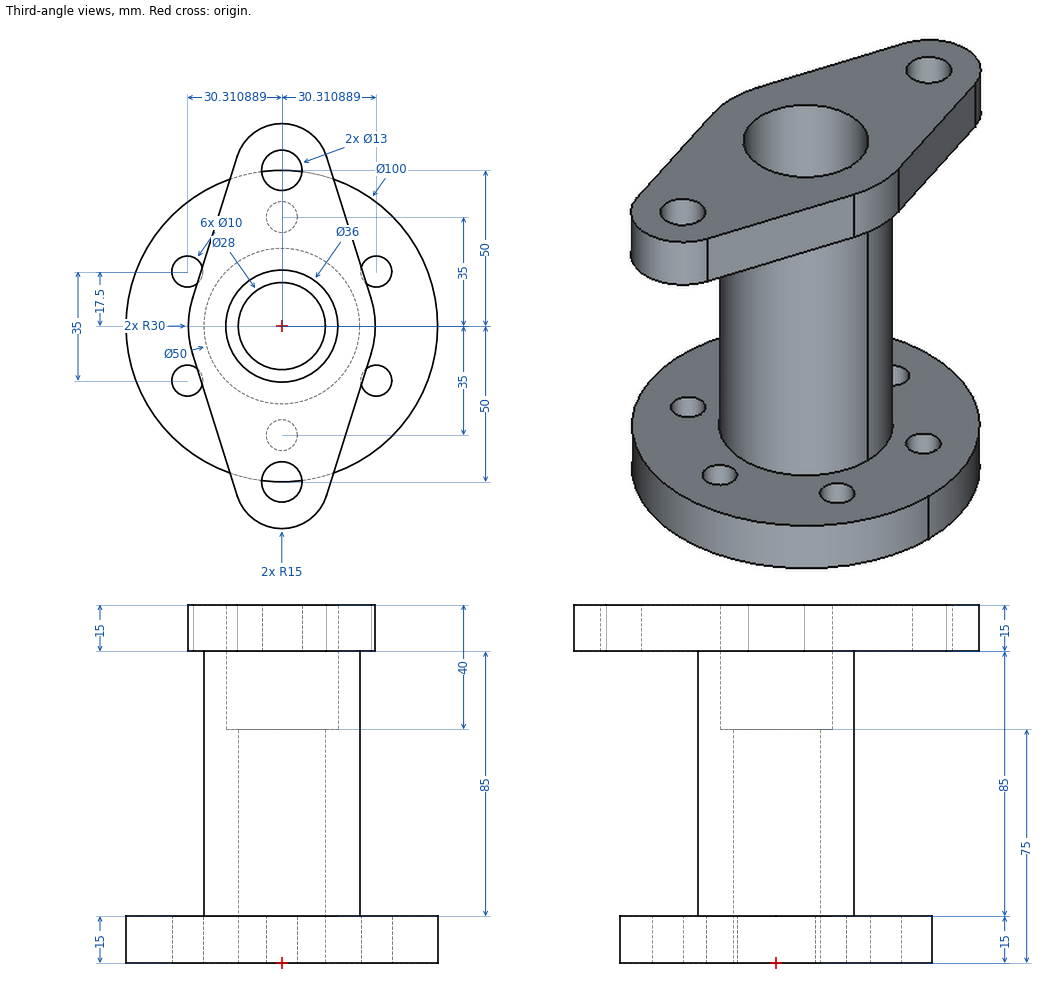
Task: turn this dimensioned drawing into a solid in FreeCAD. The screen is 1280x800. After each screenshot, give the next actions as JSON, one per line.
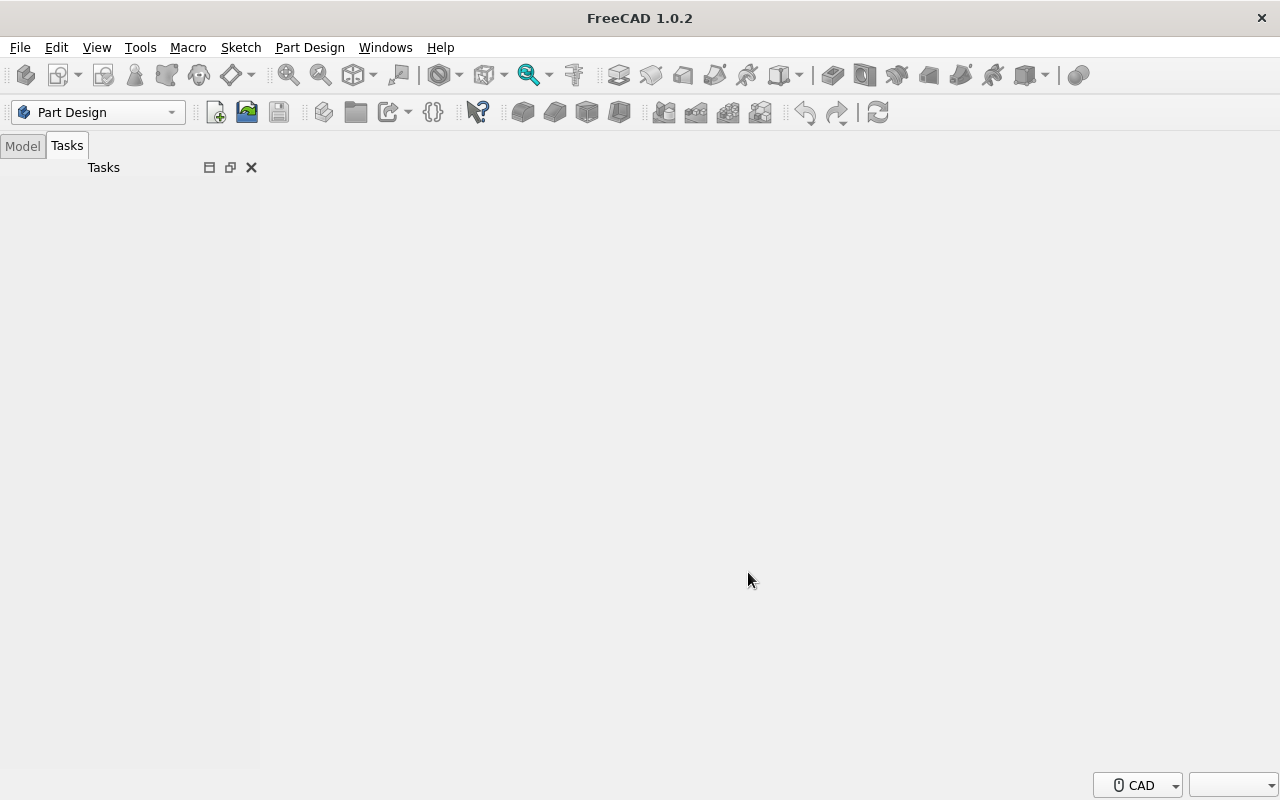
{"action": "key", "text": "ctrl+n"}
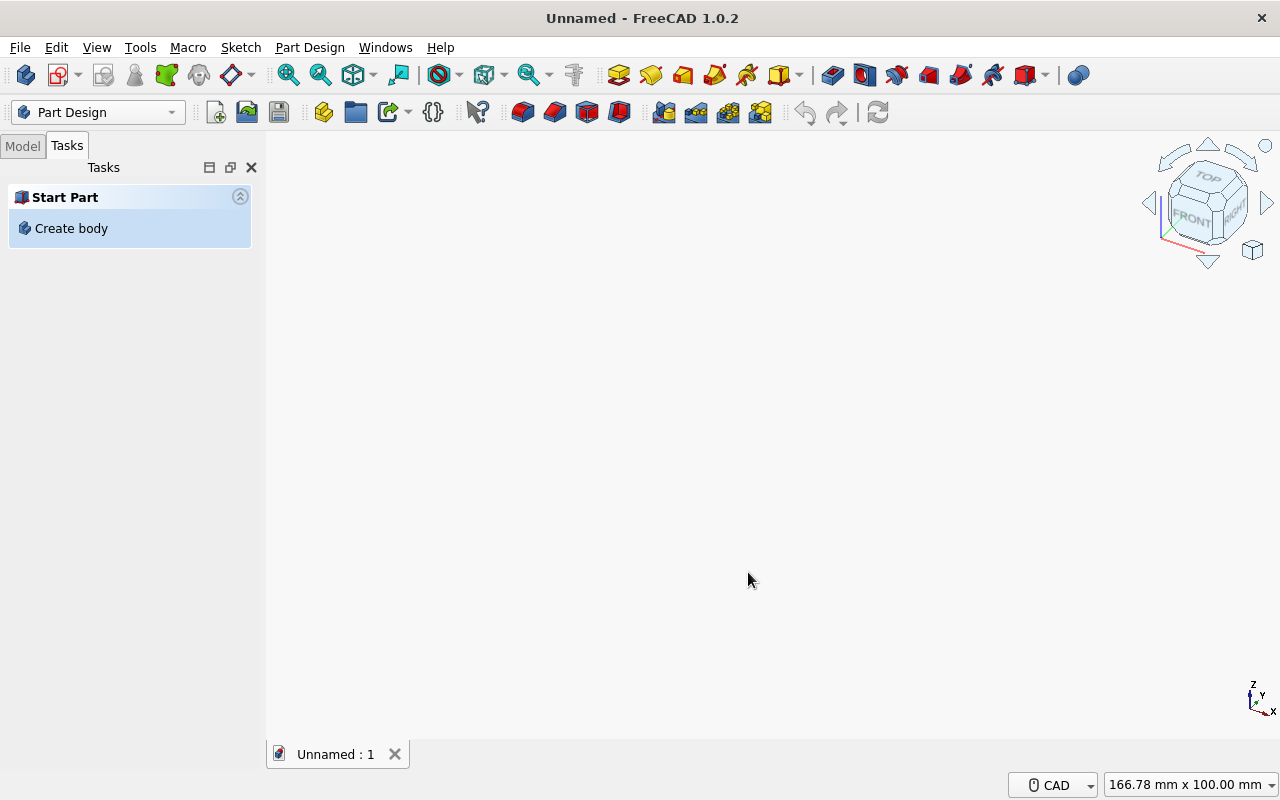
{"action": "left_click", "coordinate": [58, 76]}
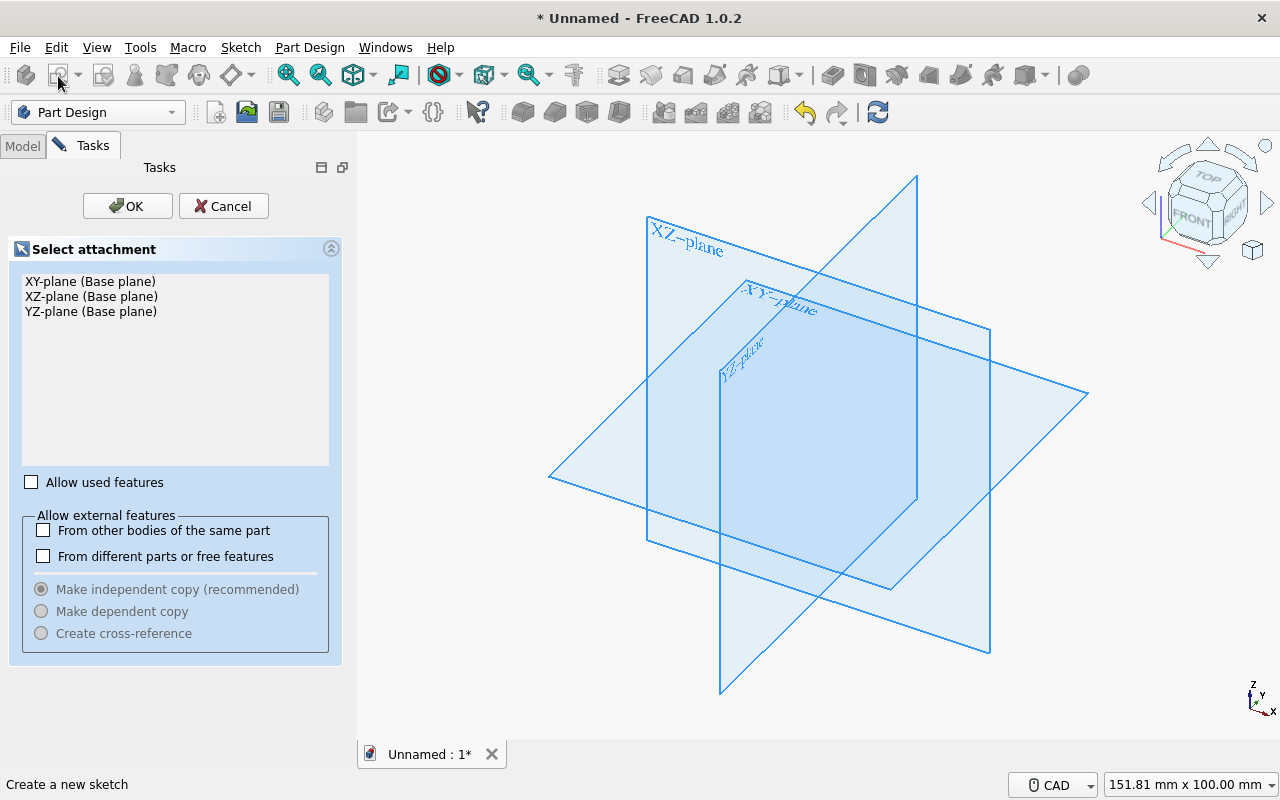
{"action": "left_click", "coordinate": [82, 282]}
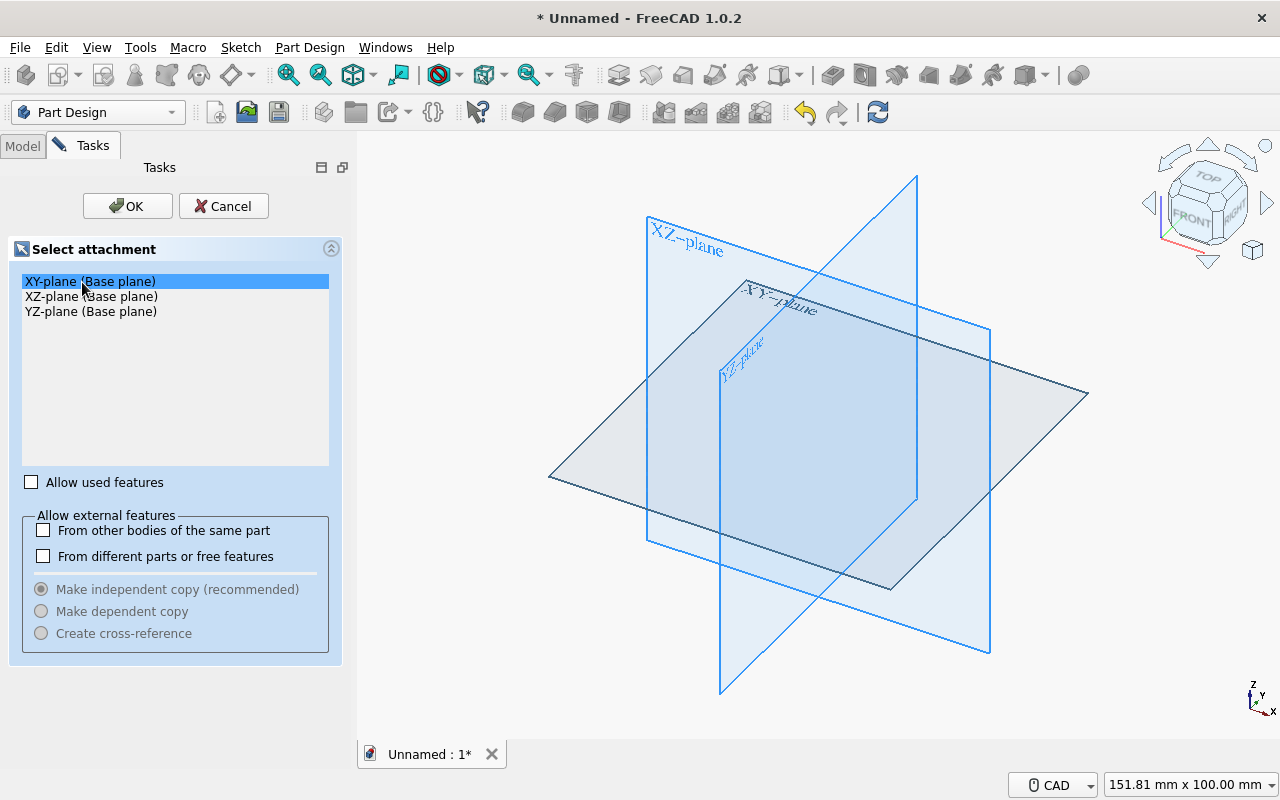
{"action": "left_click", "coordinate": [128, 206]}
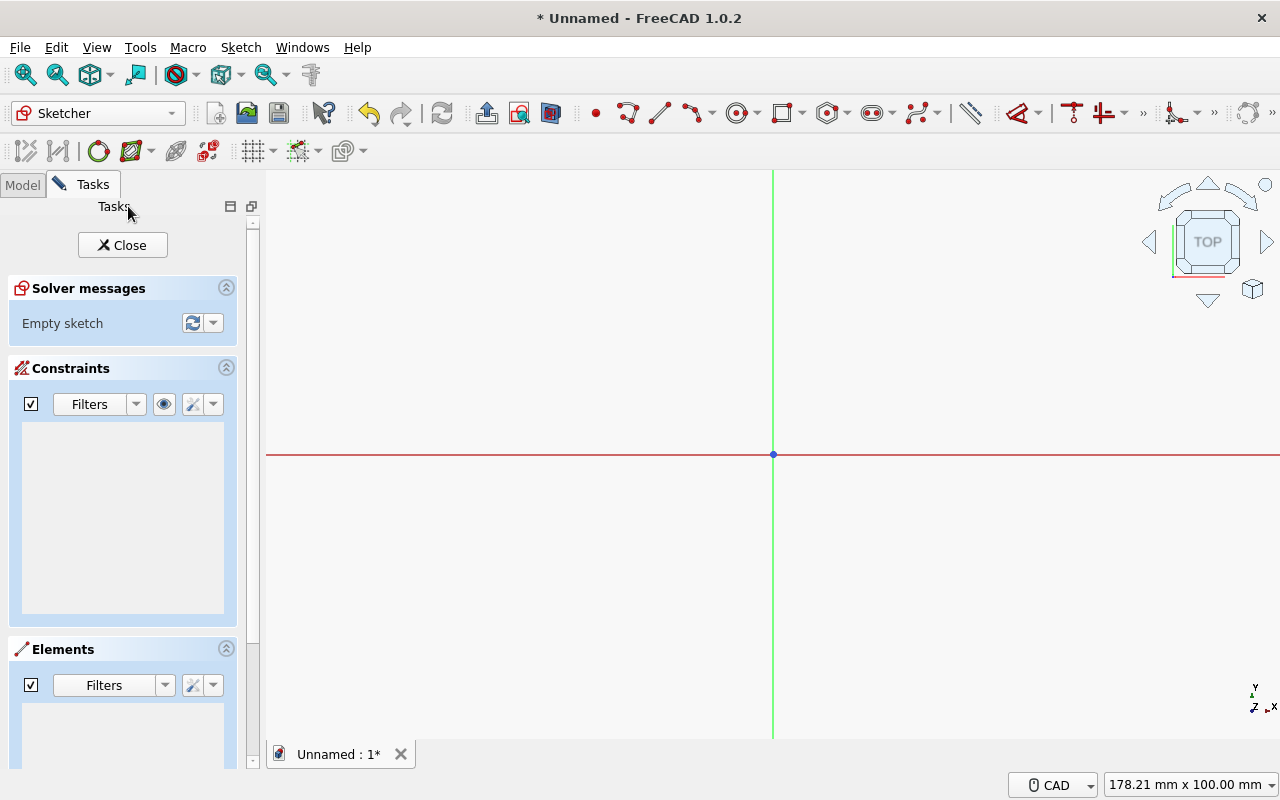
{"action": "scroll", "coordinate": [565, 455], "scroll_direction": "down", "scroll_amount": 2}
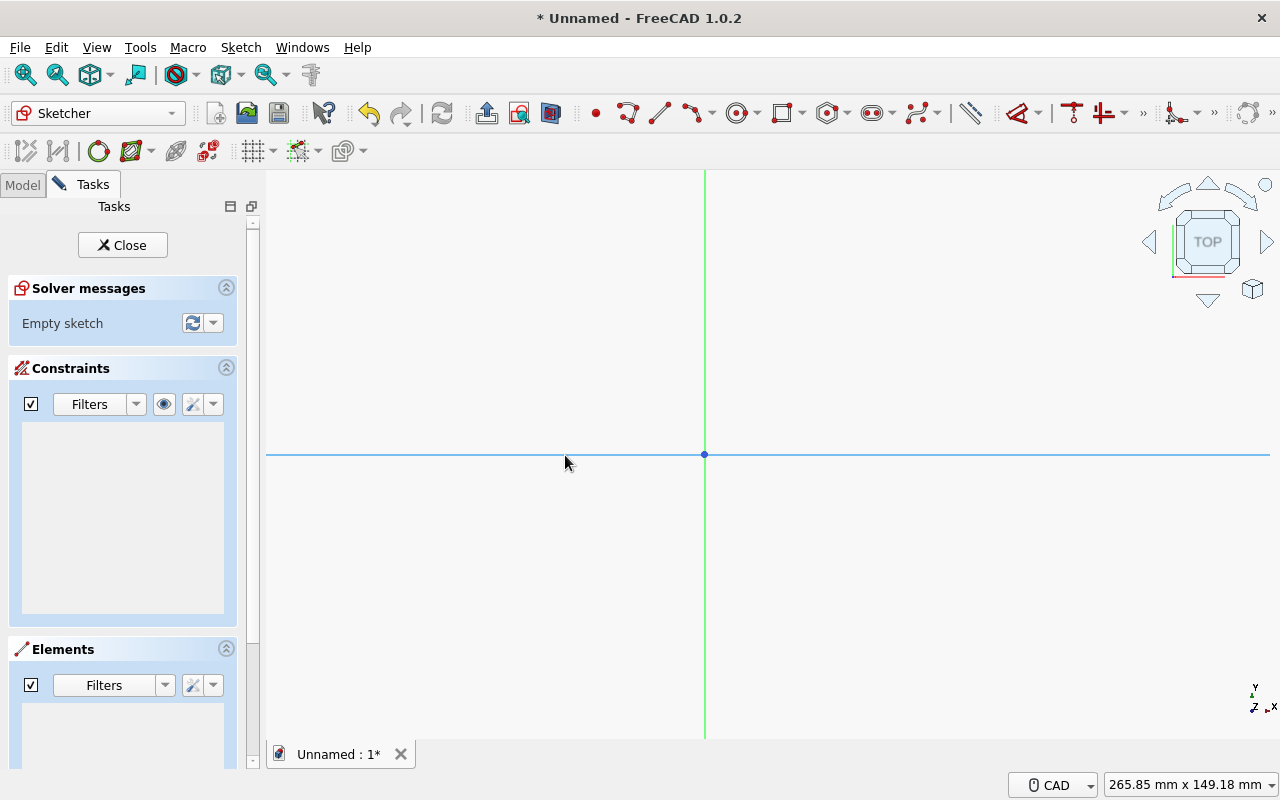
{"action": "left_click", "coordinate": [738, 114]}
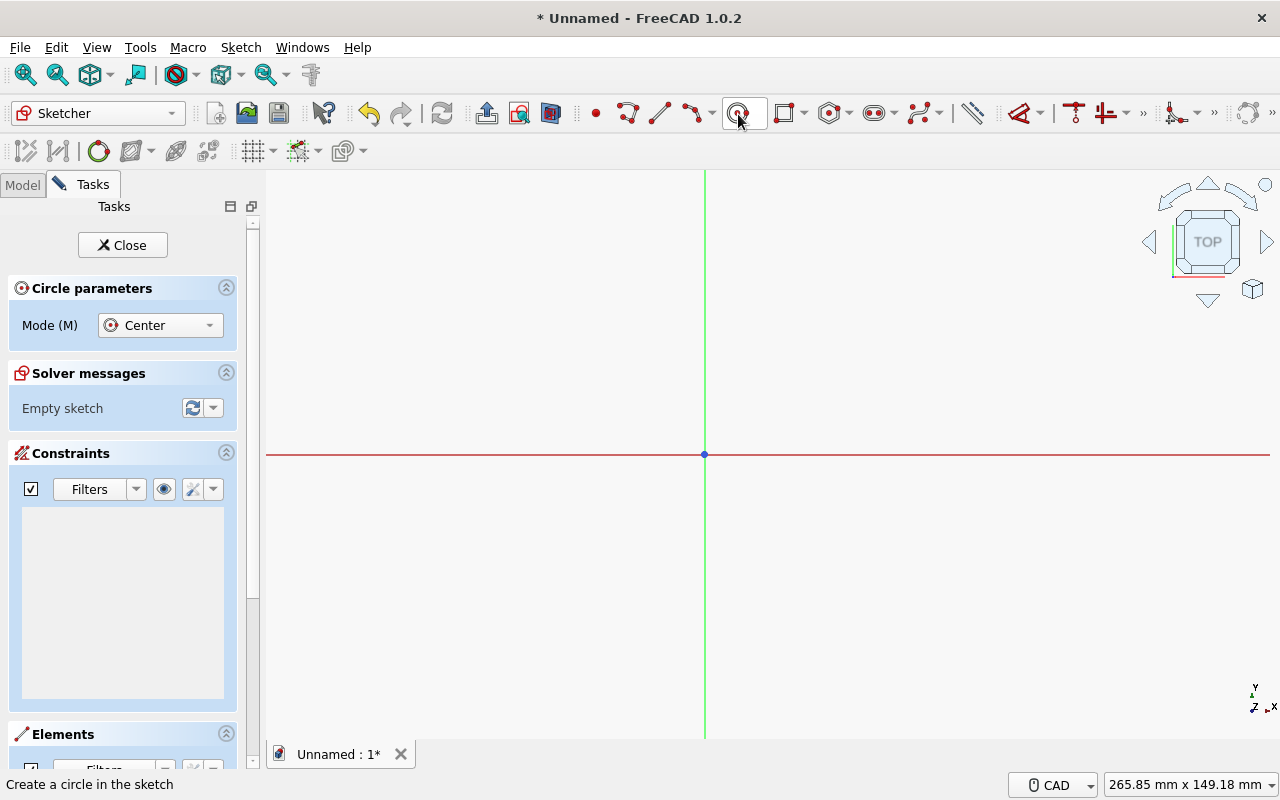
{"action": "left_click", "coordinate": [705, 455]}
{"action": "mouse_move", "coordinate": [839, 320]}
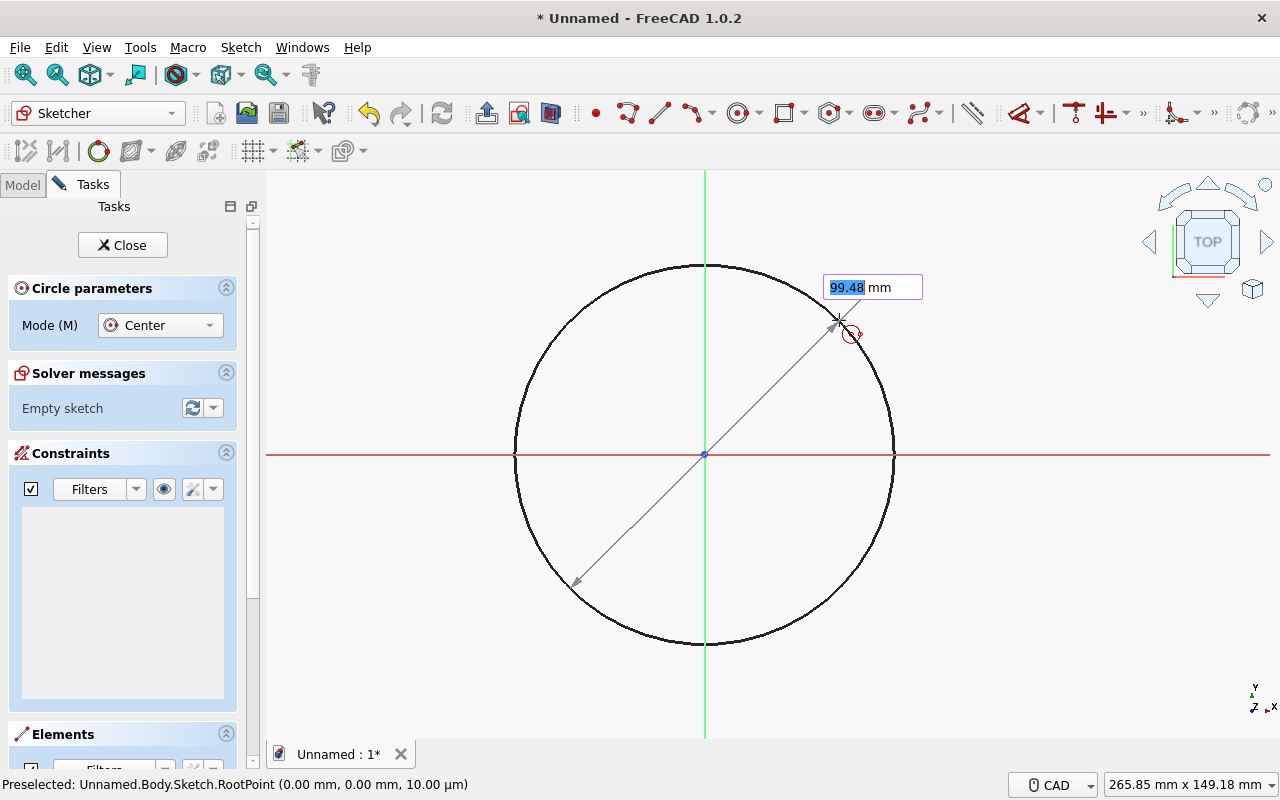
{"action": "type", "text": "100"}
{"action": "key", "text": "Return"}
{"action": "key", "text": "Escape"}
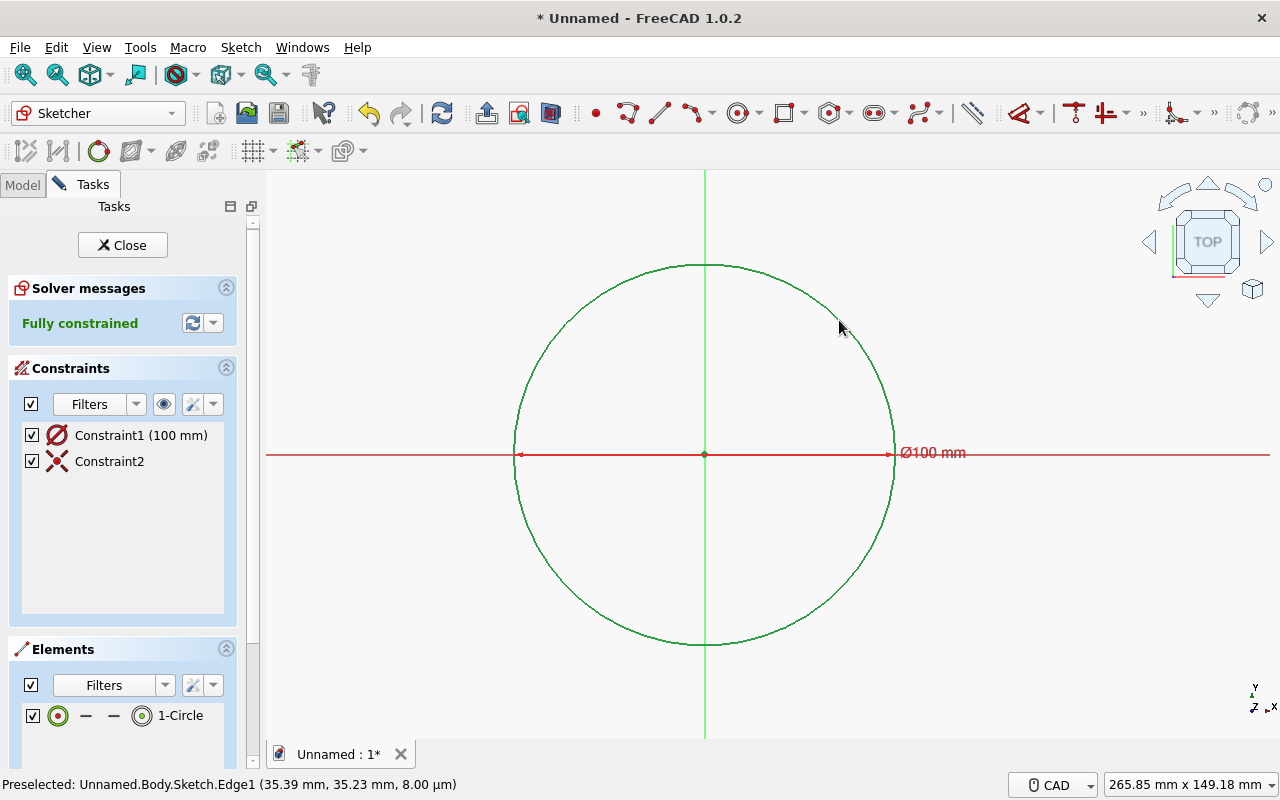
{"action": "left_click", "coordinate": [123, 245]}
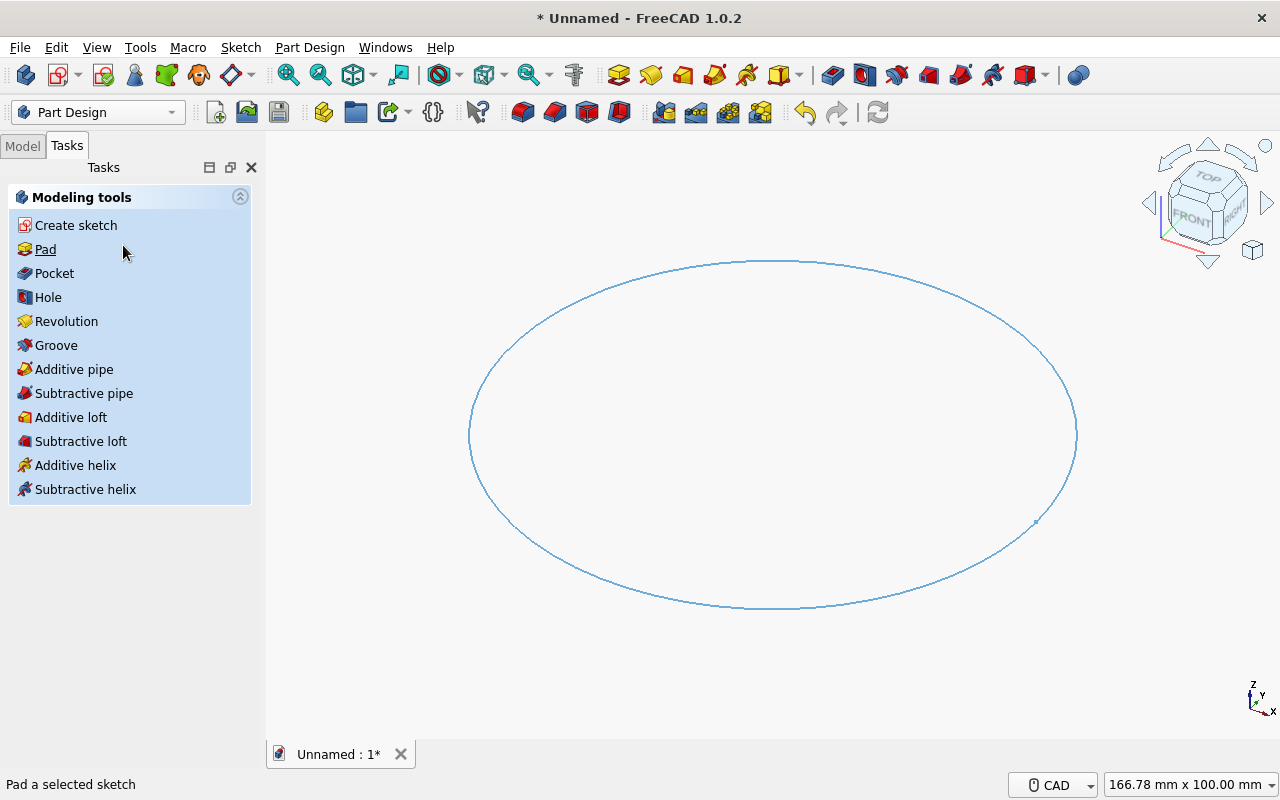
{"action": "left_click", "coordinate": [620, 76]}